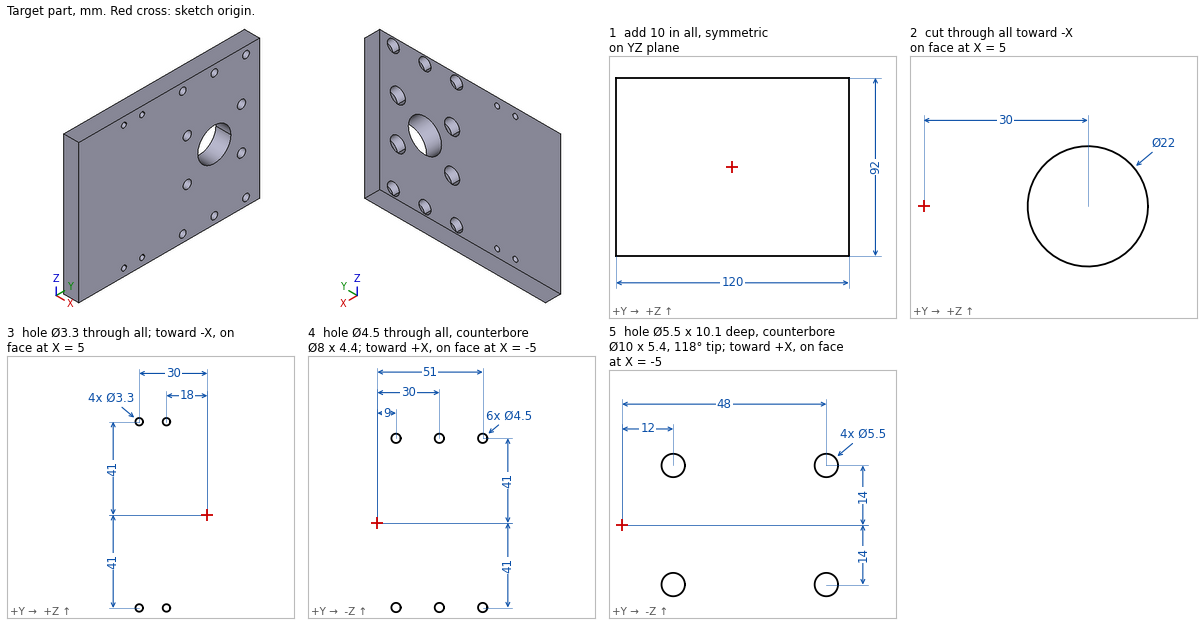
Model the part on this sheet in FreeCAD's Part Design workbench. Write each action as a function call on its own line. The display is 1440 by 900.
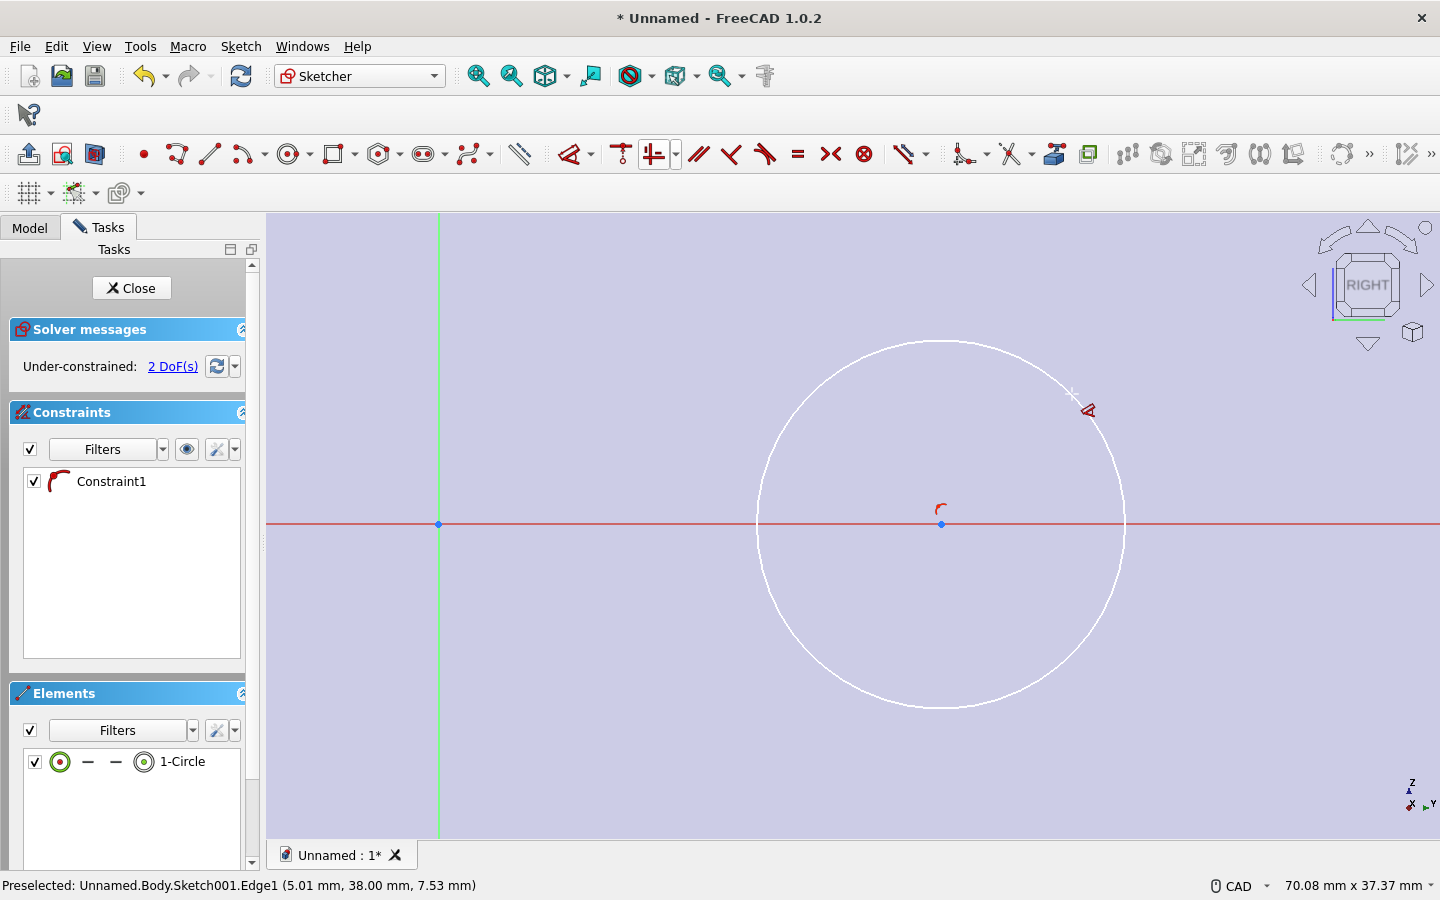
click(1071, 394)
click(1094, 371)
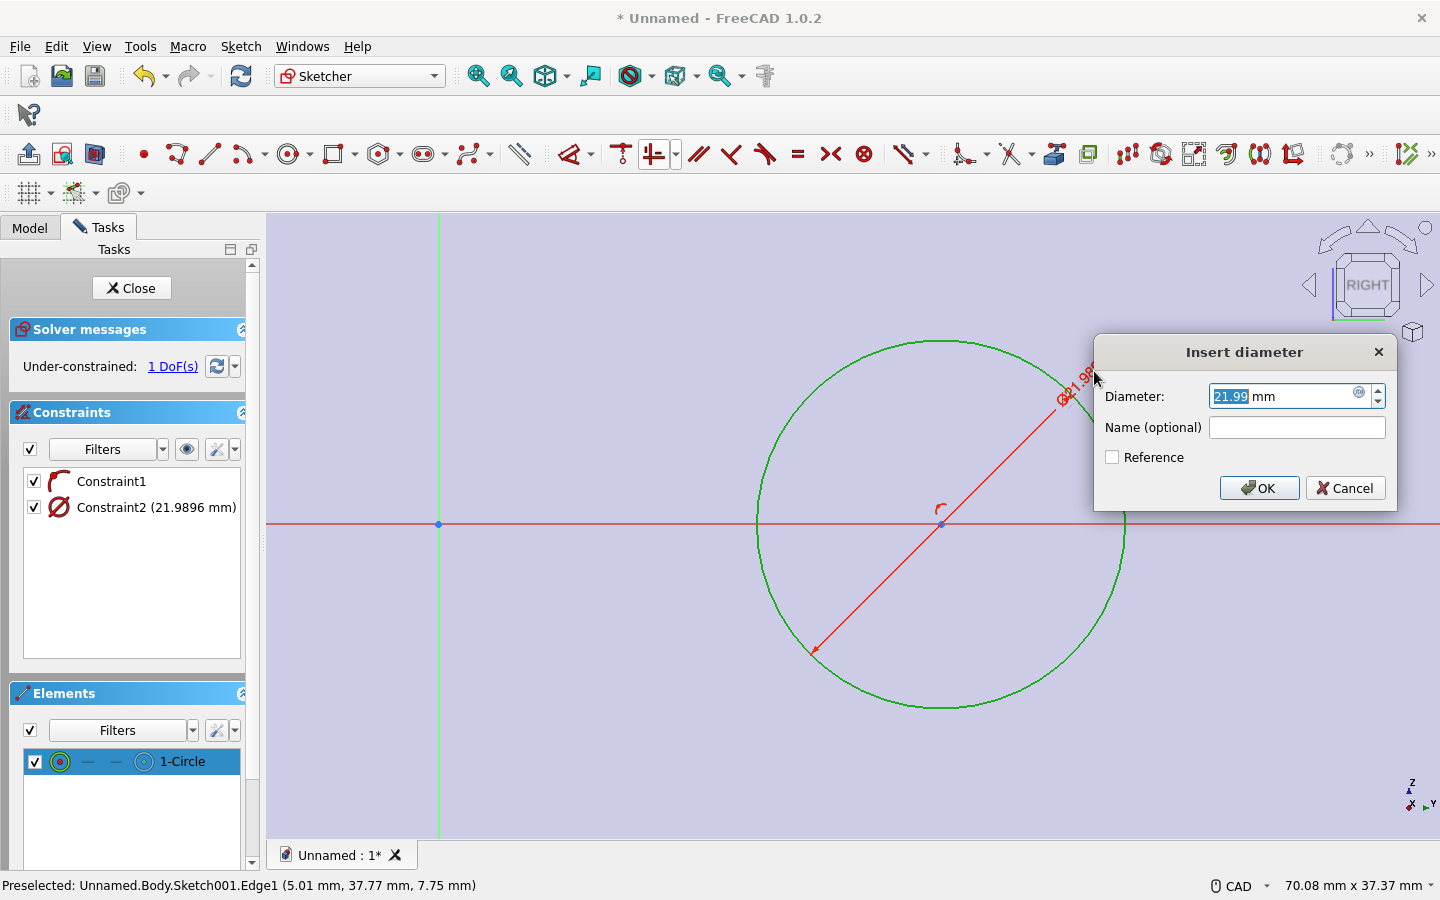
text(22)
key(Return)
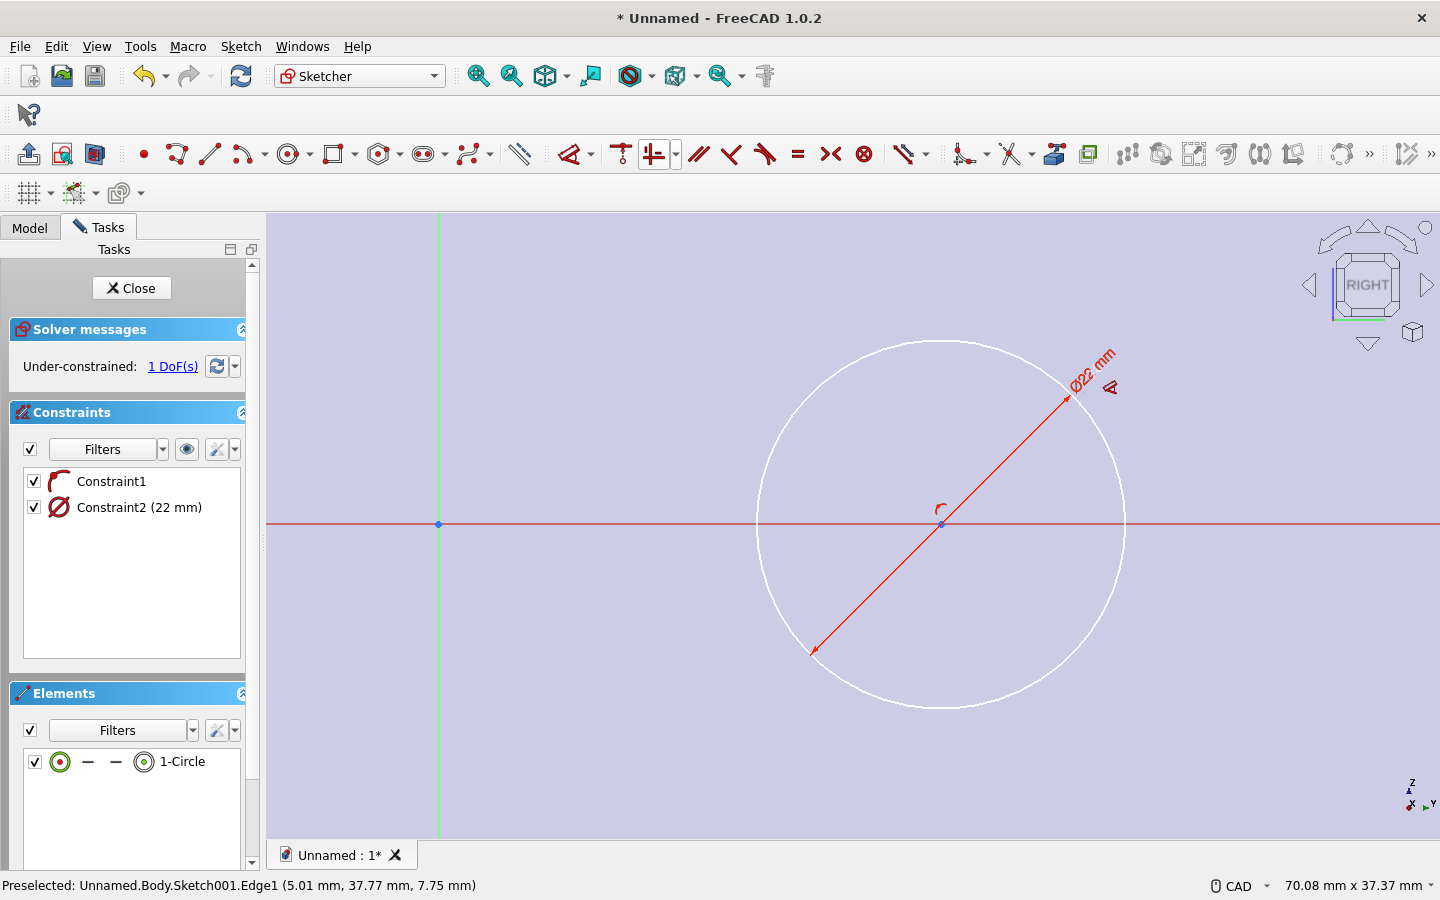
click(941, 524)
click(690, 558)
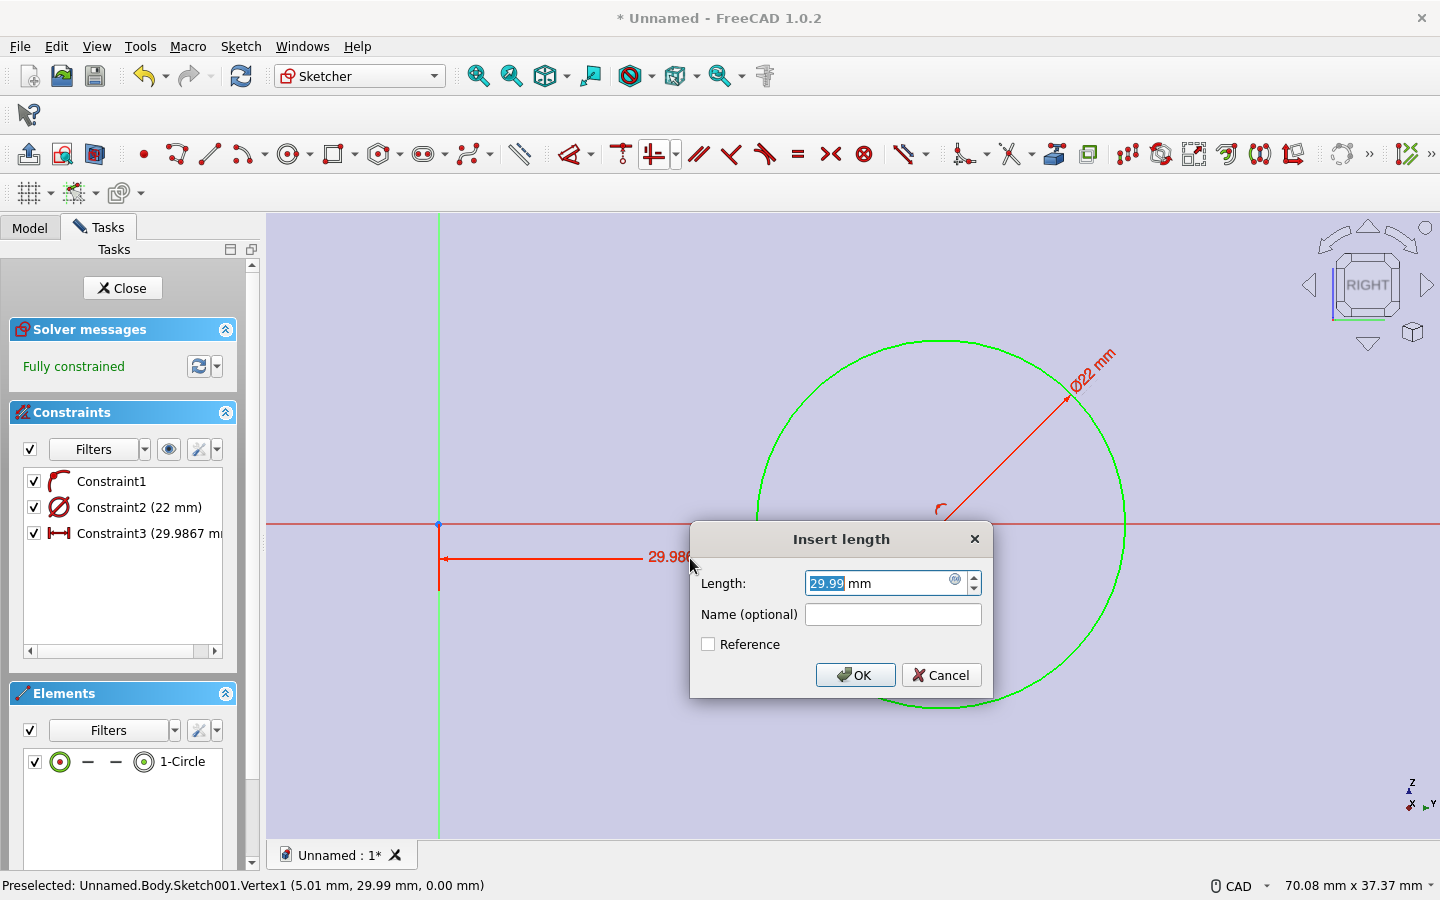
text(30)
key(Return)
key(Escape)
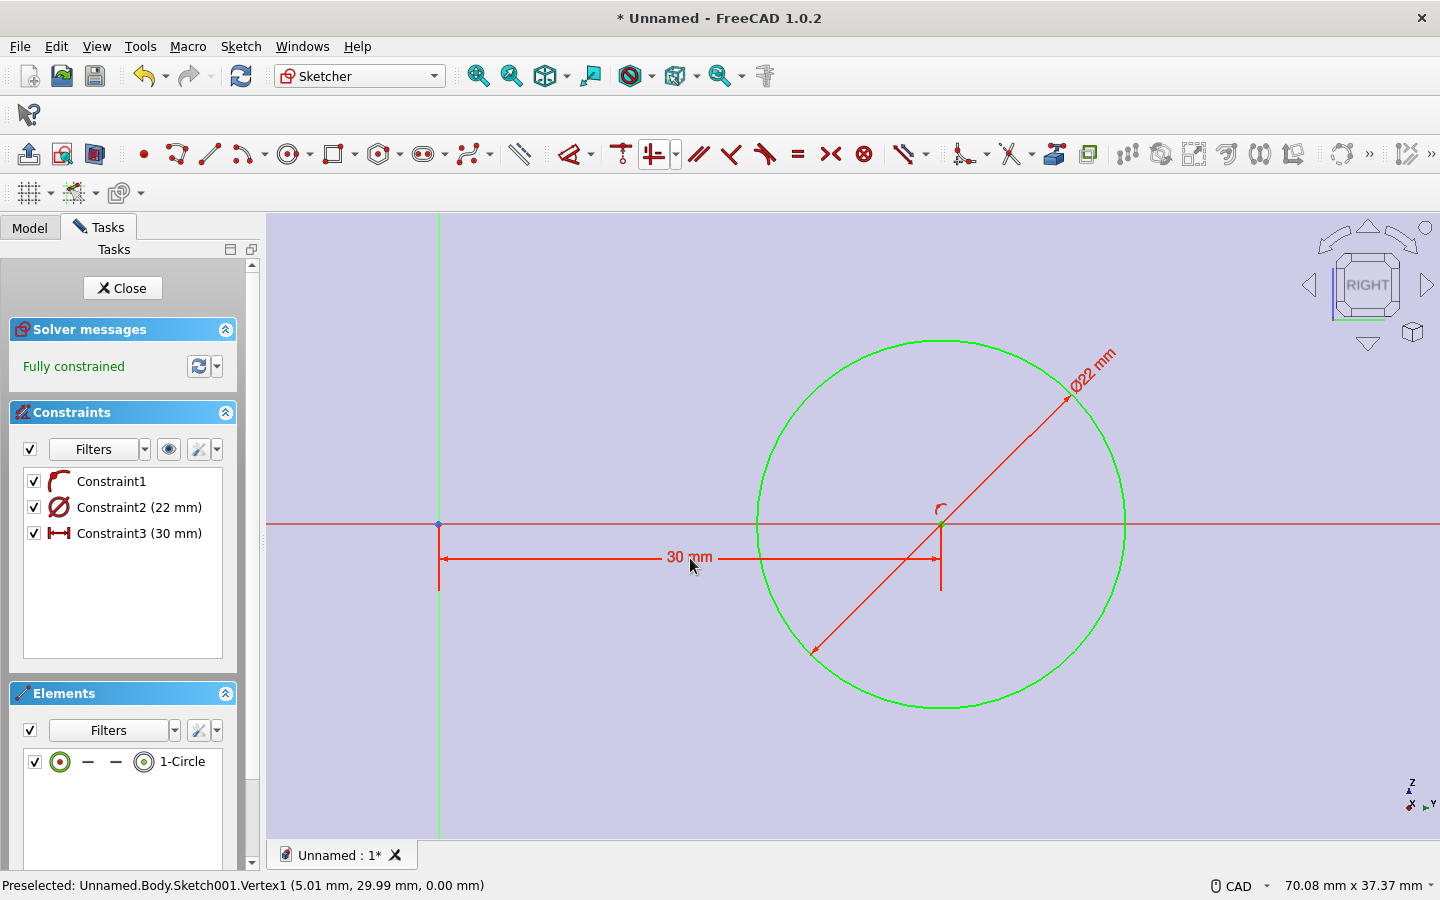
click(123, 288)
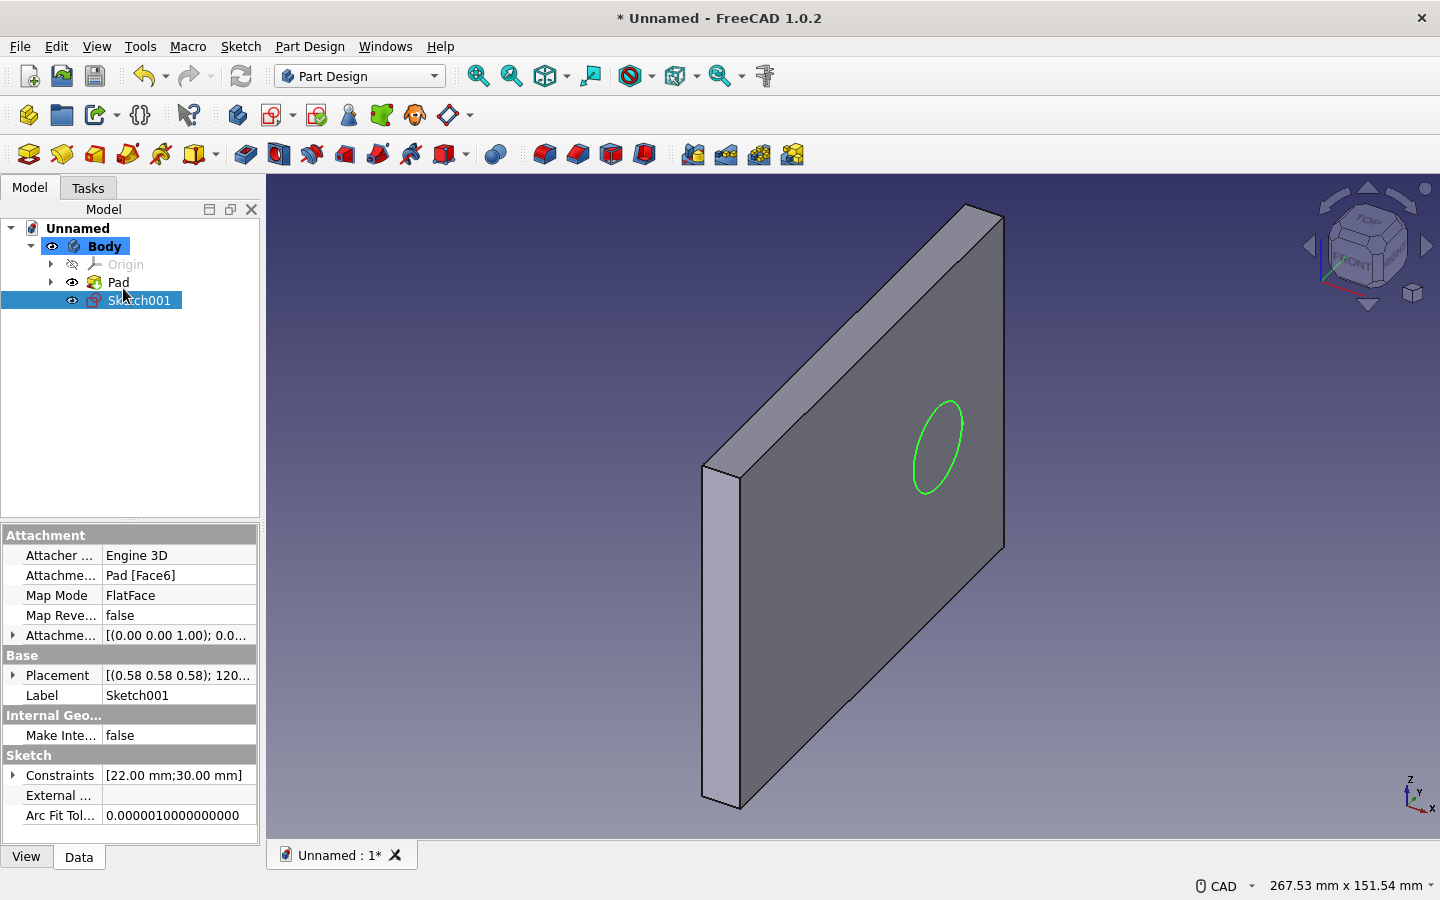
click(246, 154)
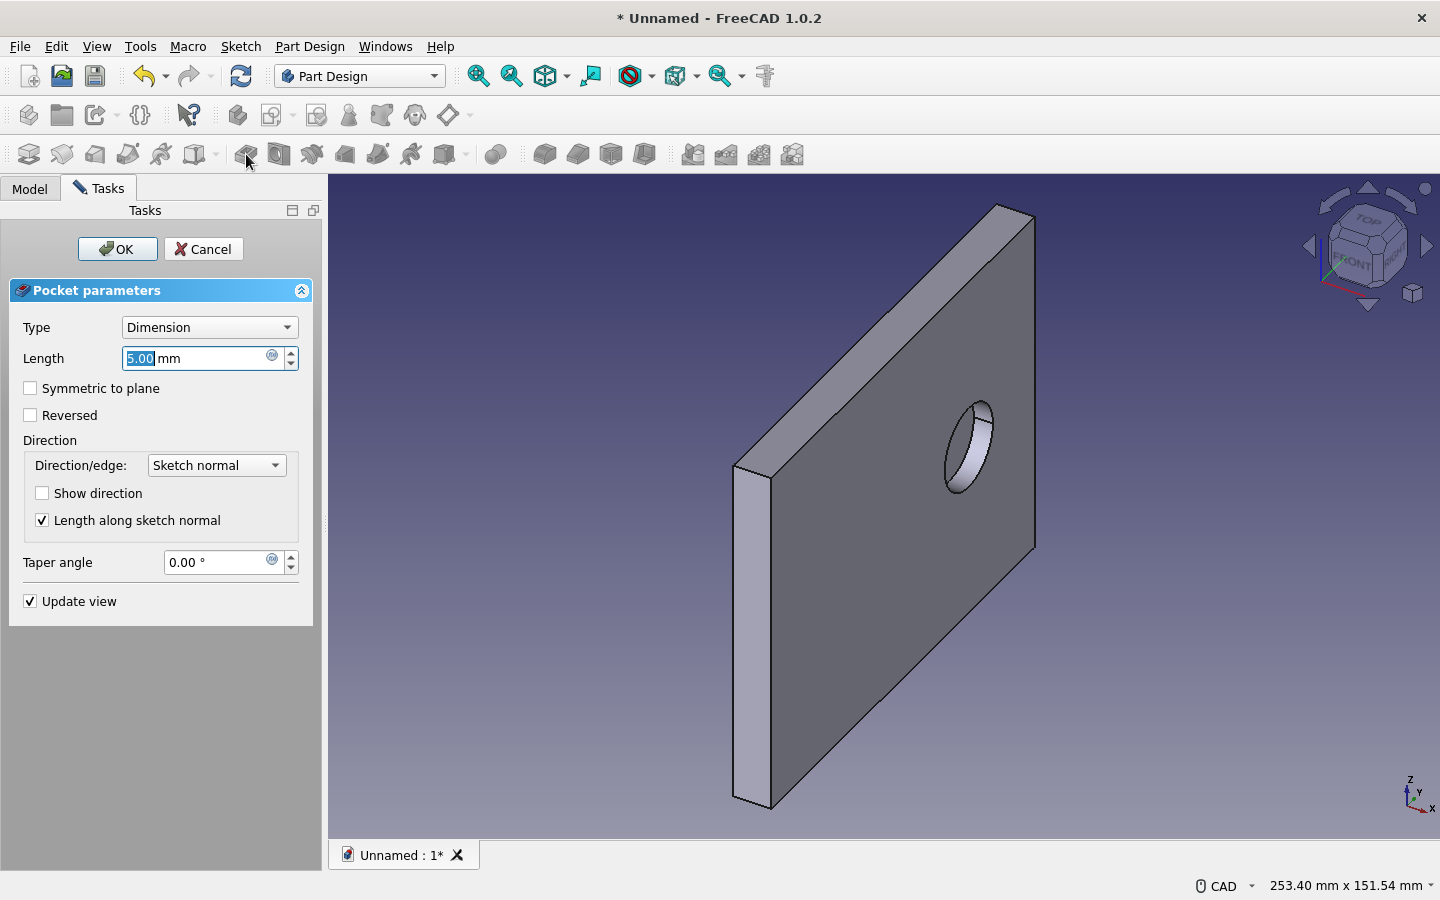
click(210, 328)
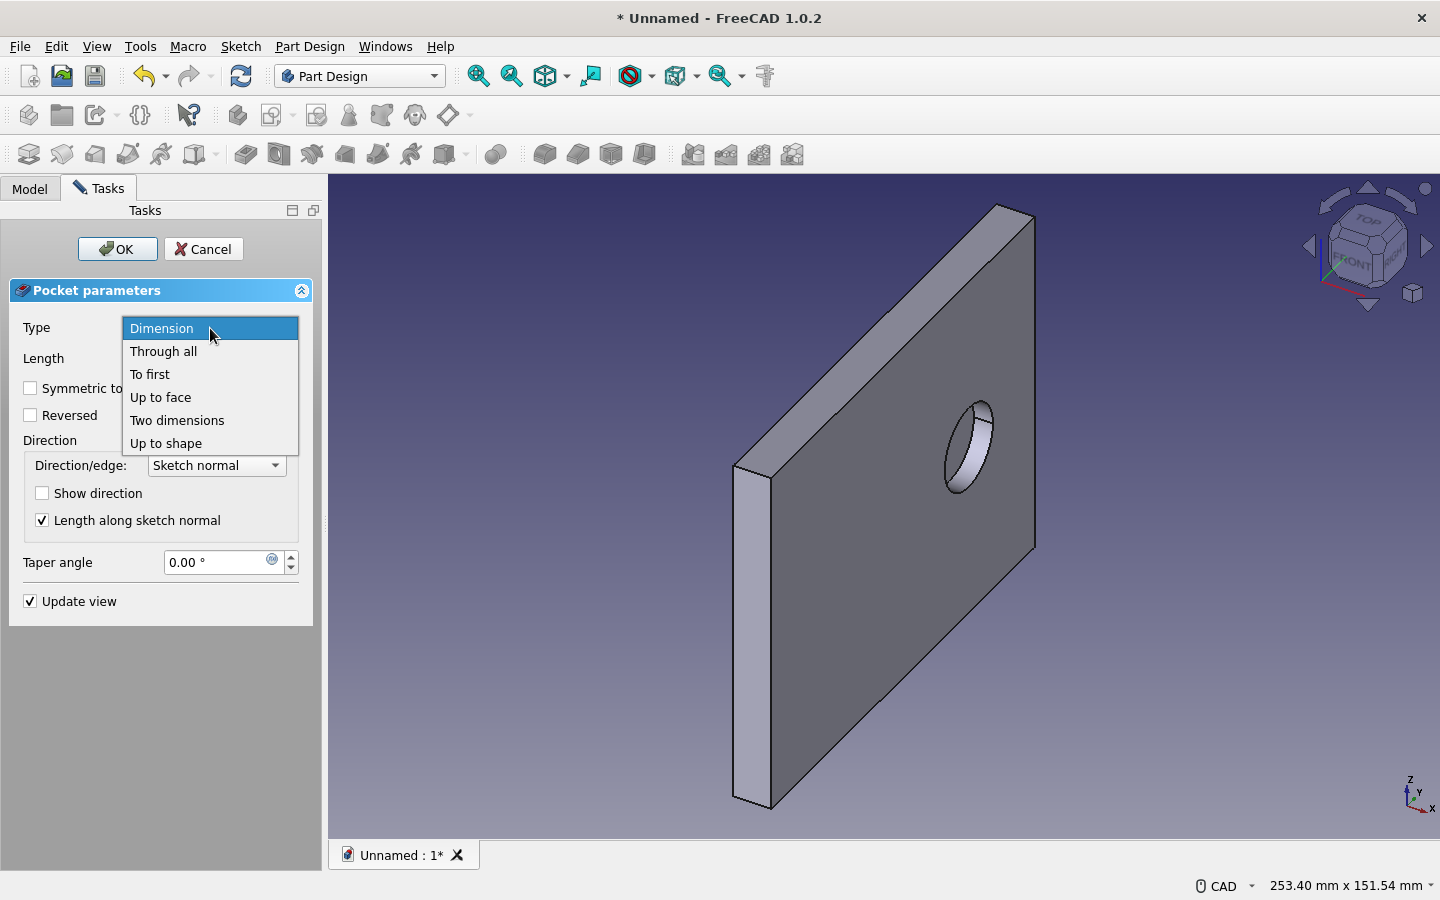
click(208, 352)